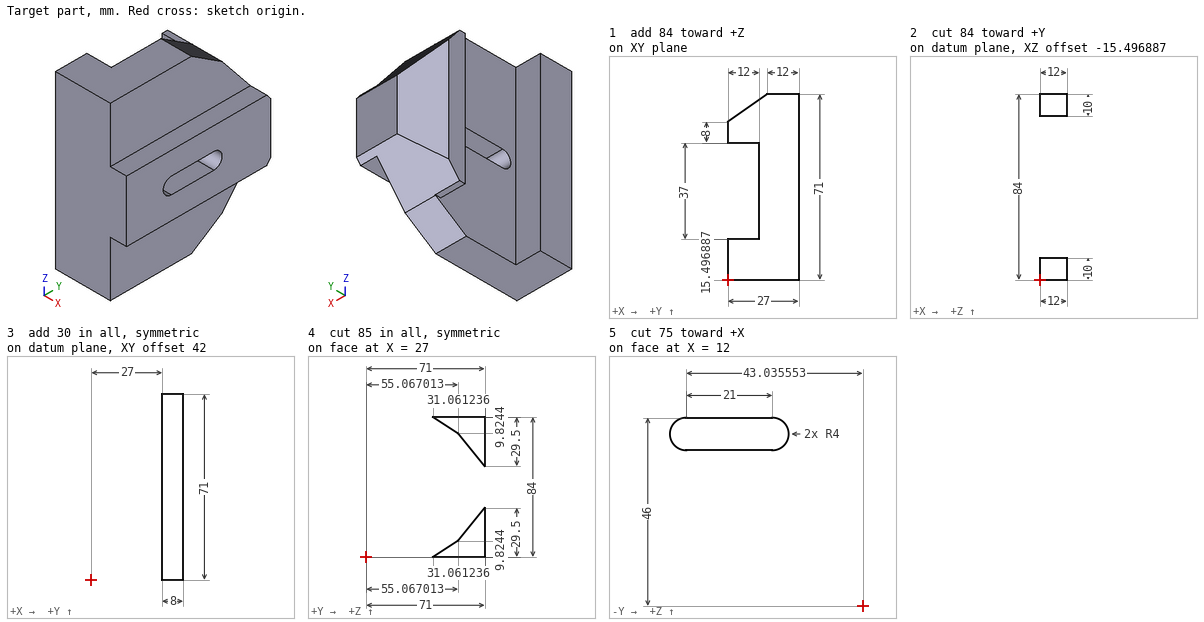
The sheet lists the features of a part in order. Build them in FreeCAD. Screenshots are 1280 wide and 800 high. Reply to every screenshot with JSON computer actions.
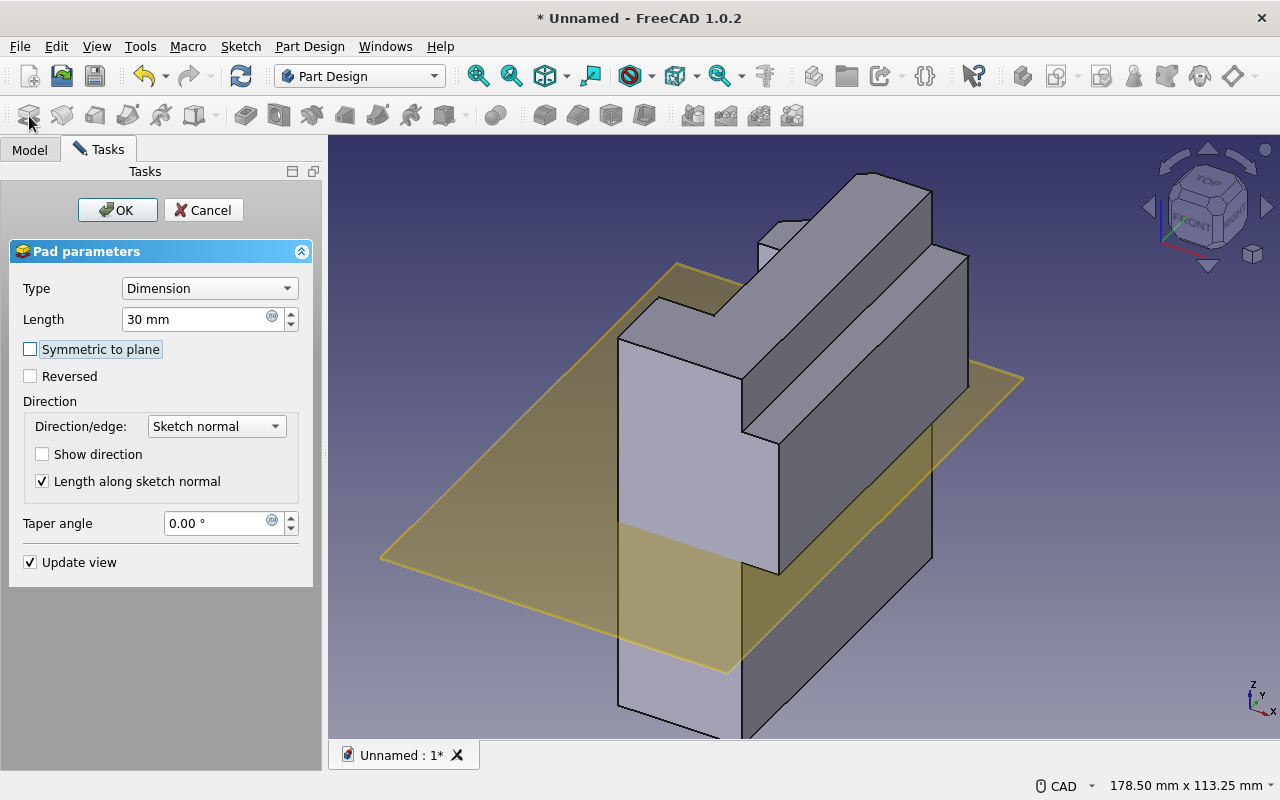
{"action": "left_click", "coordinate": [31, 349]}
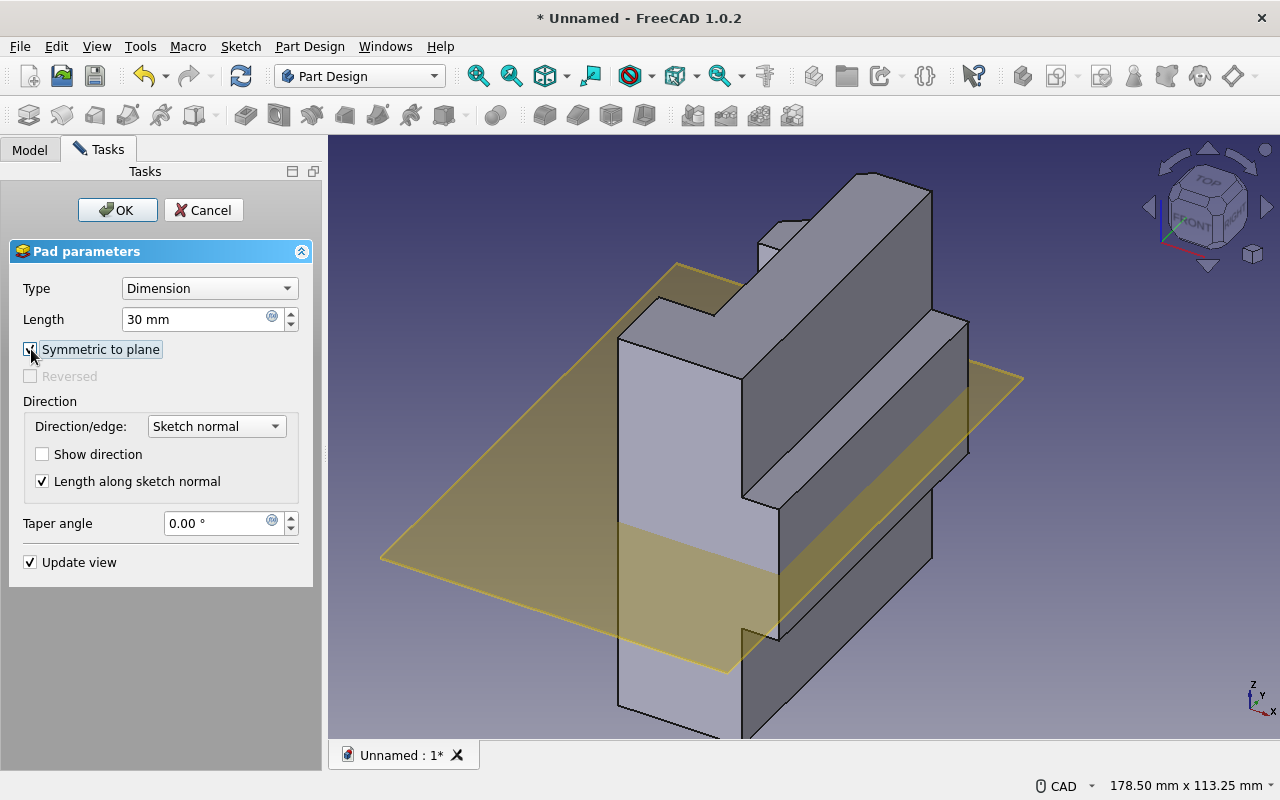
{"action": "left_click", "coordinate": [118, 210]}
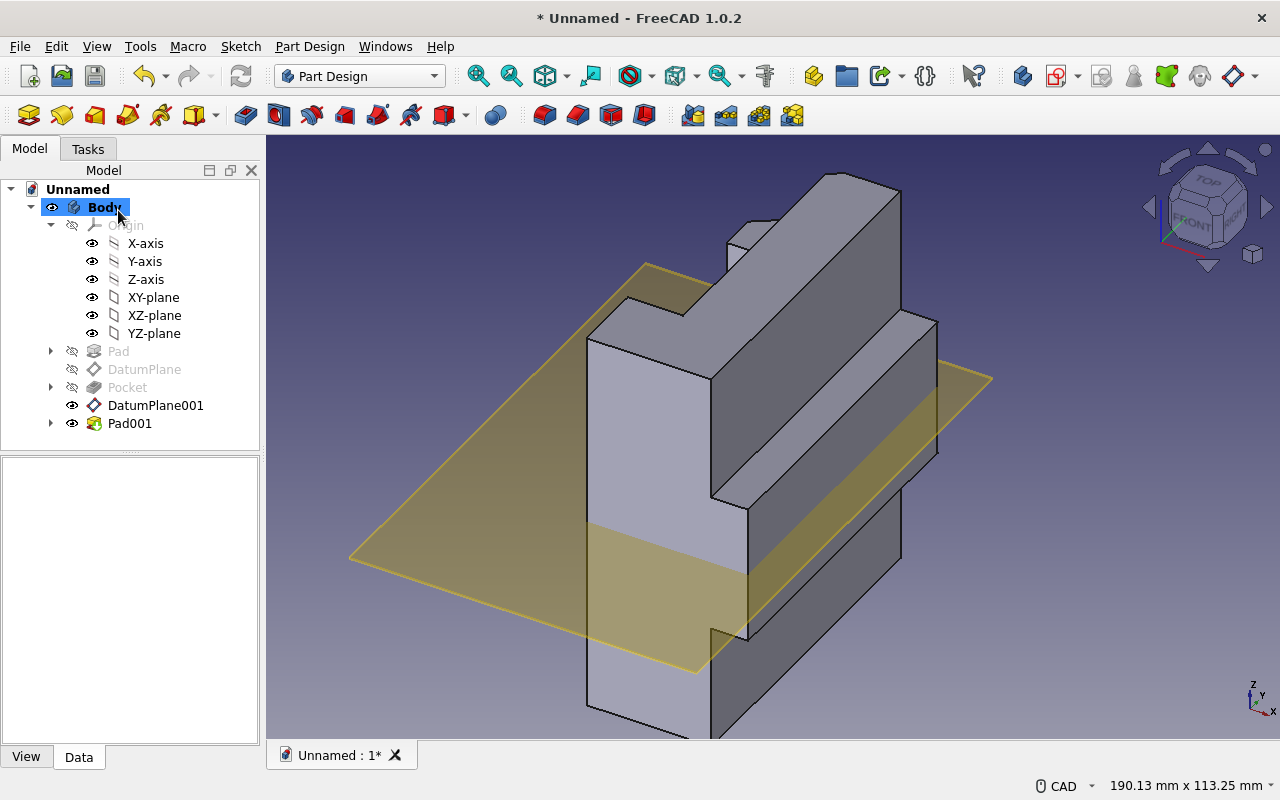
{"action": "left_click", "coordinate": [117, 405]}
{"action": "key", "text": "space"}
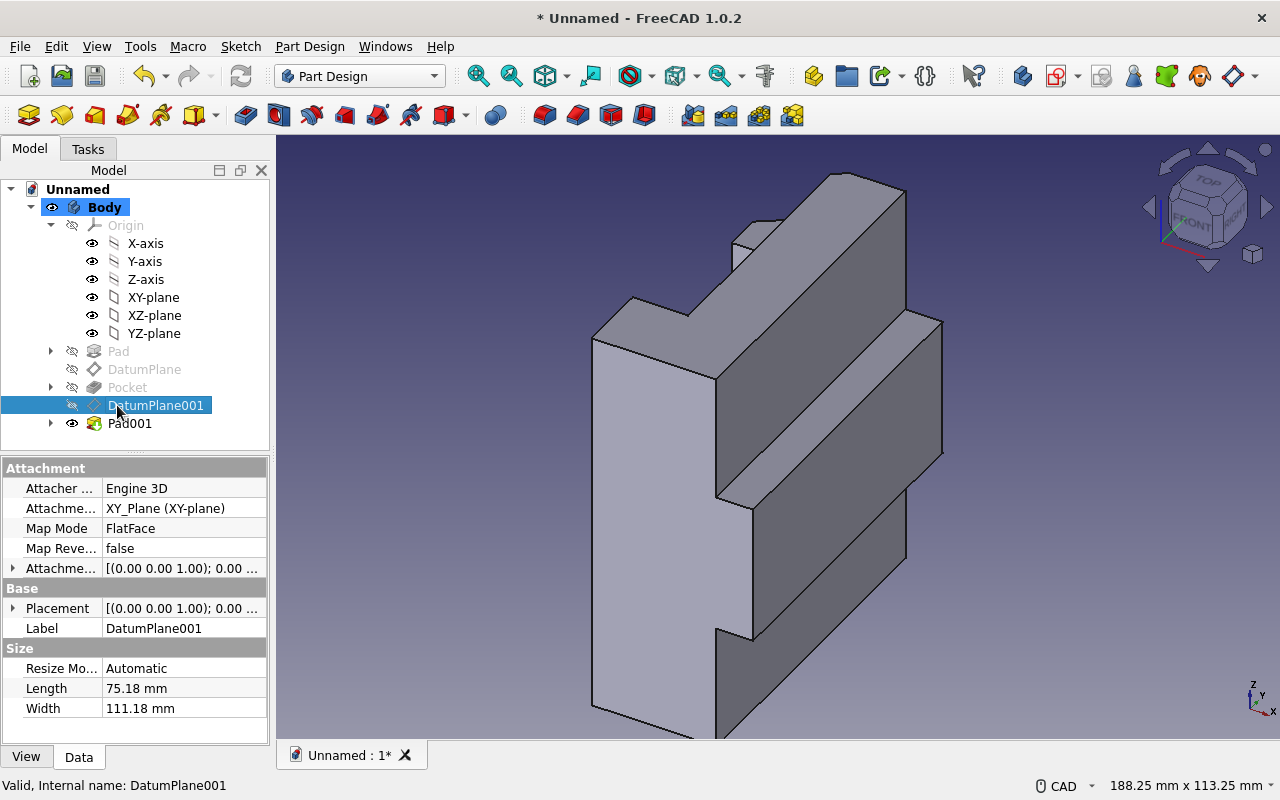
{"action": "left_click", "coordinate": [479, 76]}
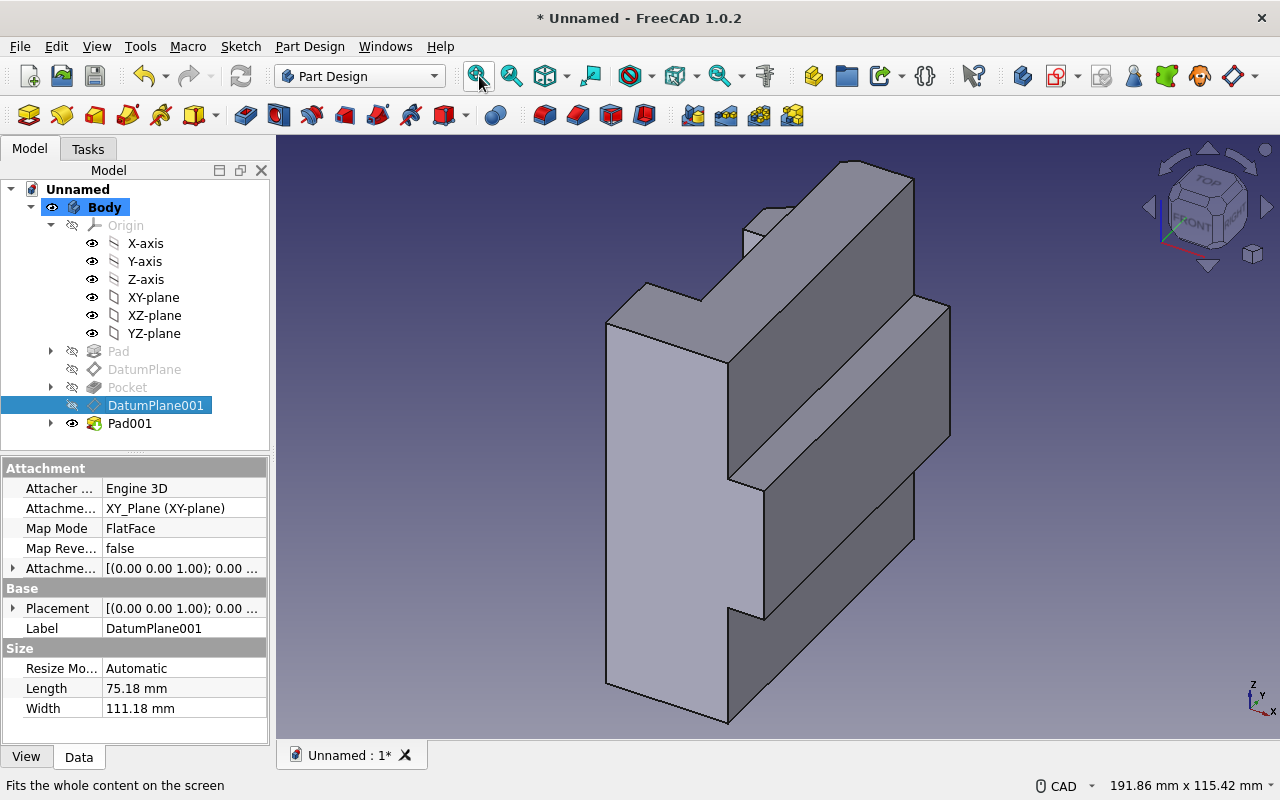
{"action": "left_click", "coordinate": [874, 275]}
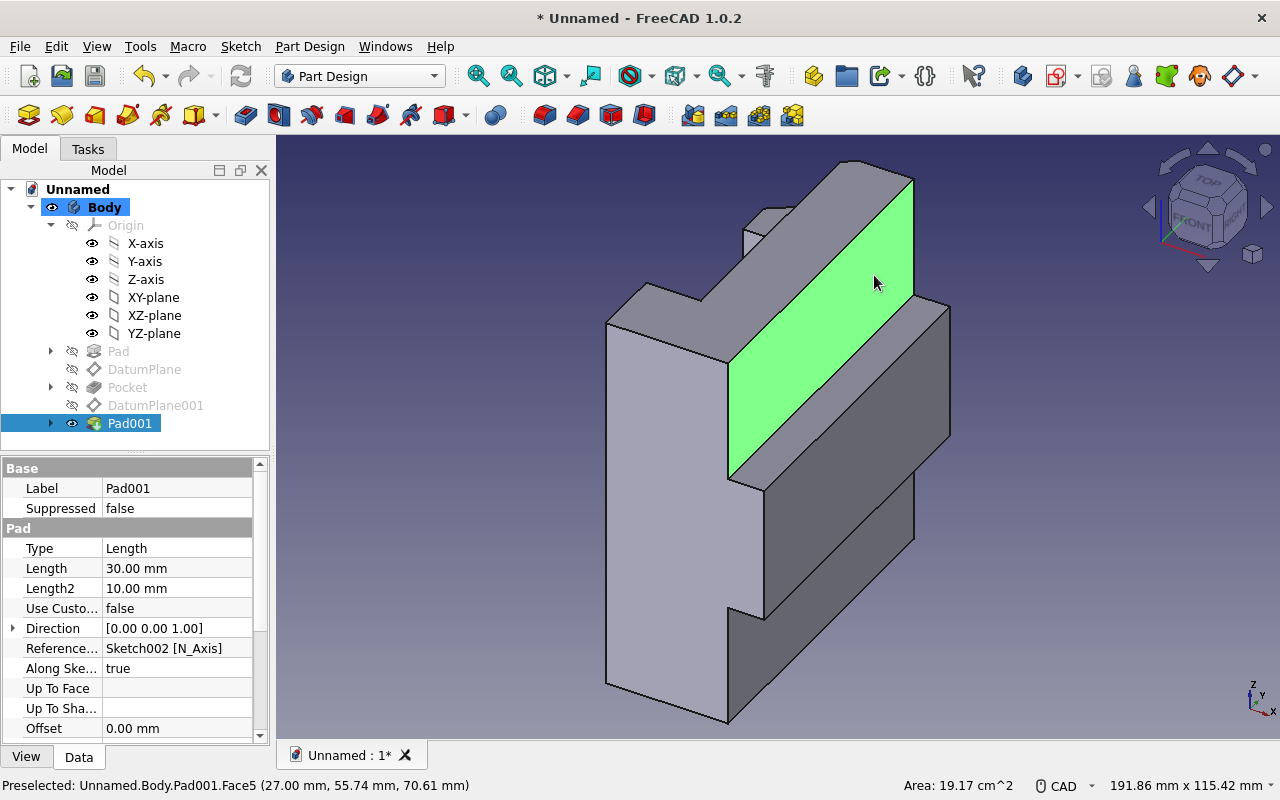
{"action": "left_click", "coordinate": [1056, 76]}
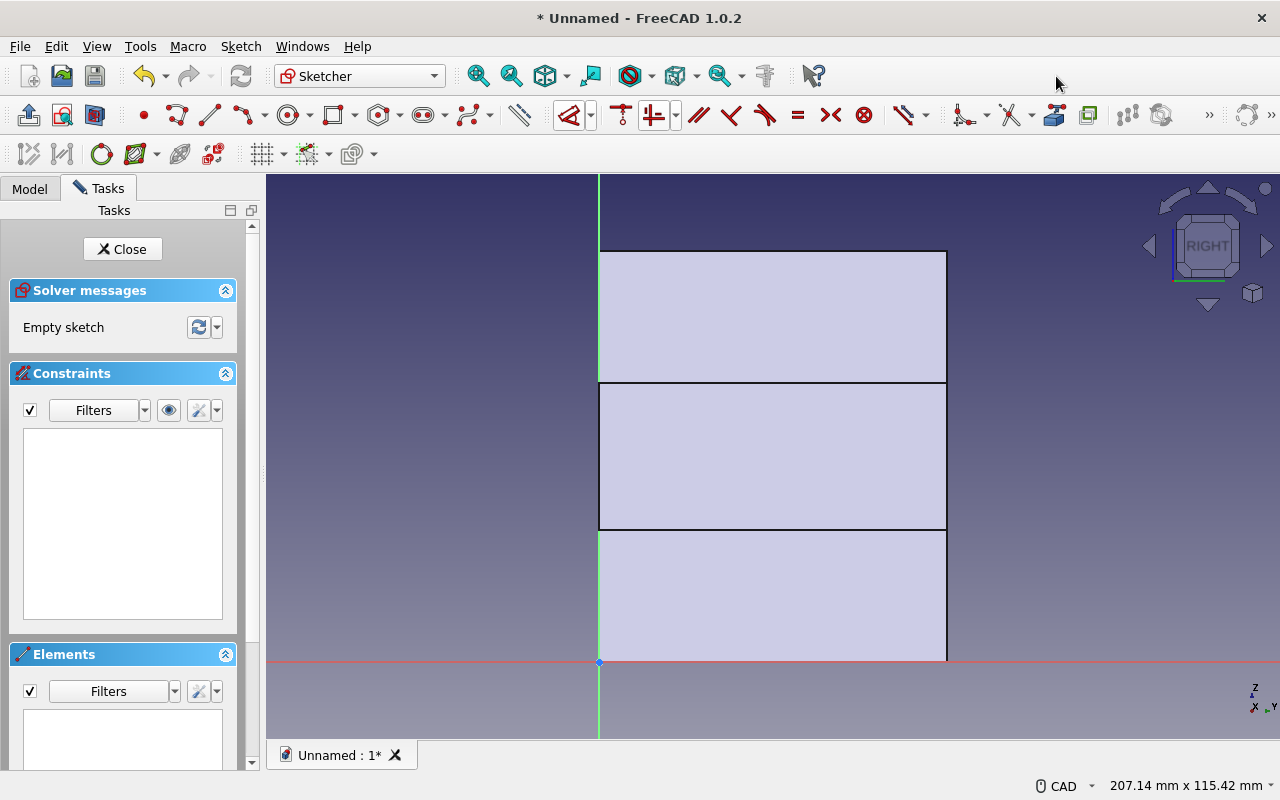
{"action": "key", "text": "q s"}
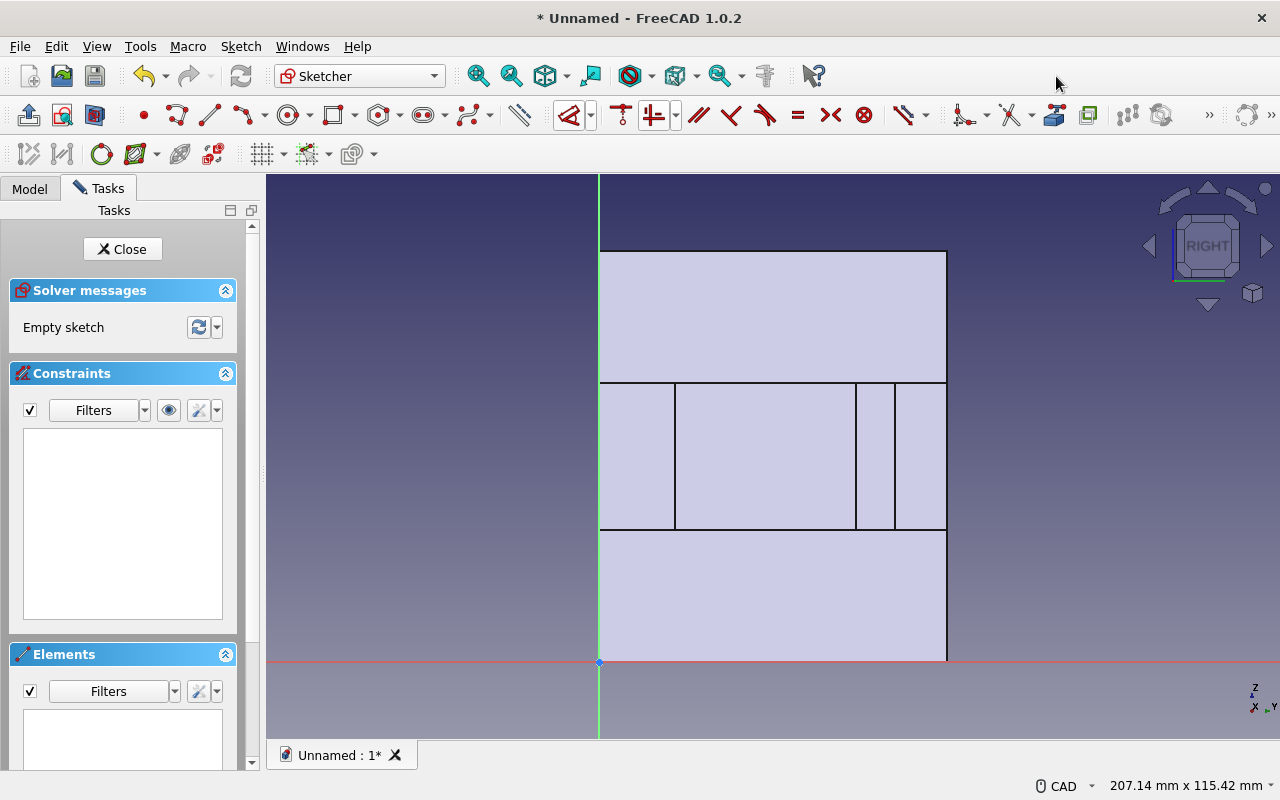
{"action": "key", "text": "g m"}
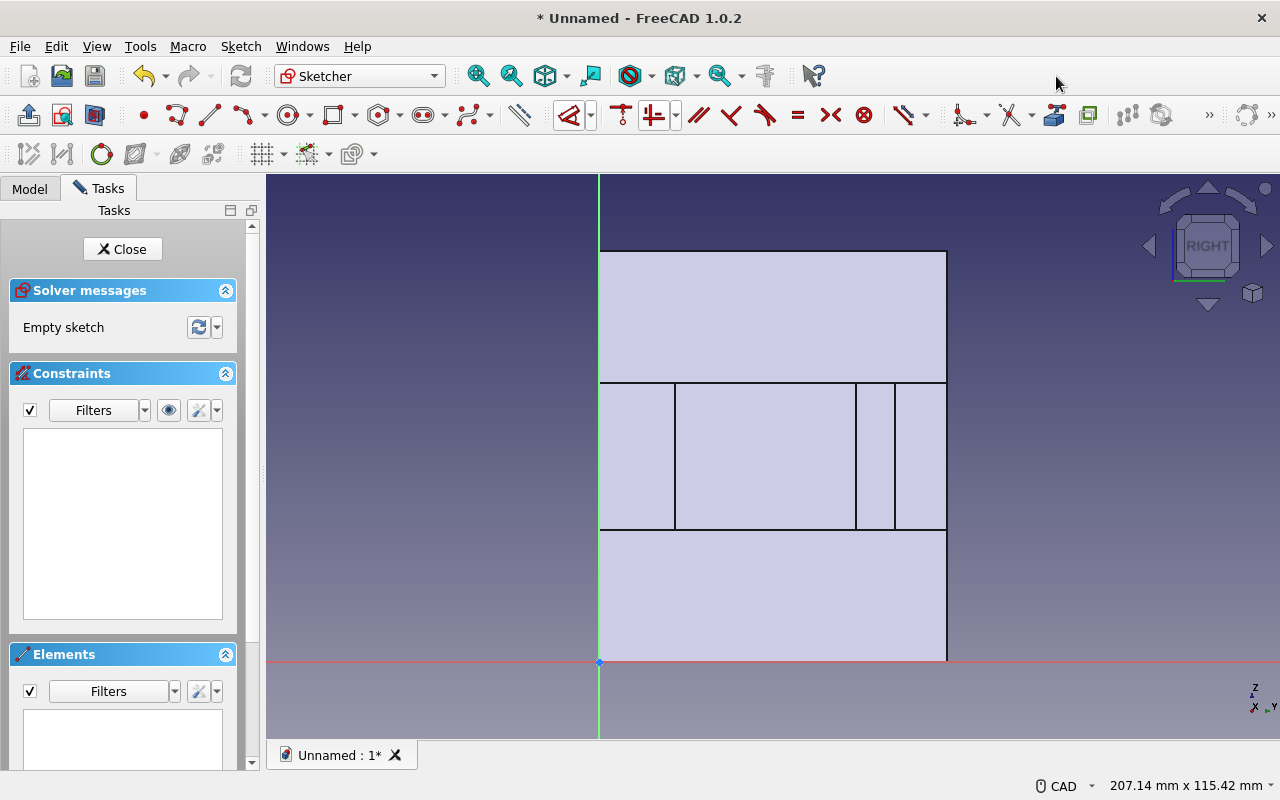
{"action": "left_click", "coordinate": [947, 395]}
{"action": "left_click", "coordinate": [947, 251]}
{"action": "left_click", "coordinate": [795, 251]}
{"action": "left_click", "coordinate": [869, 299]}
{"action": "left_click", "coordinate": [947, 396]}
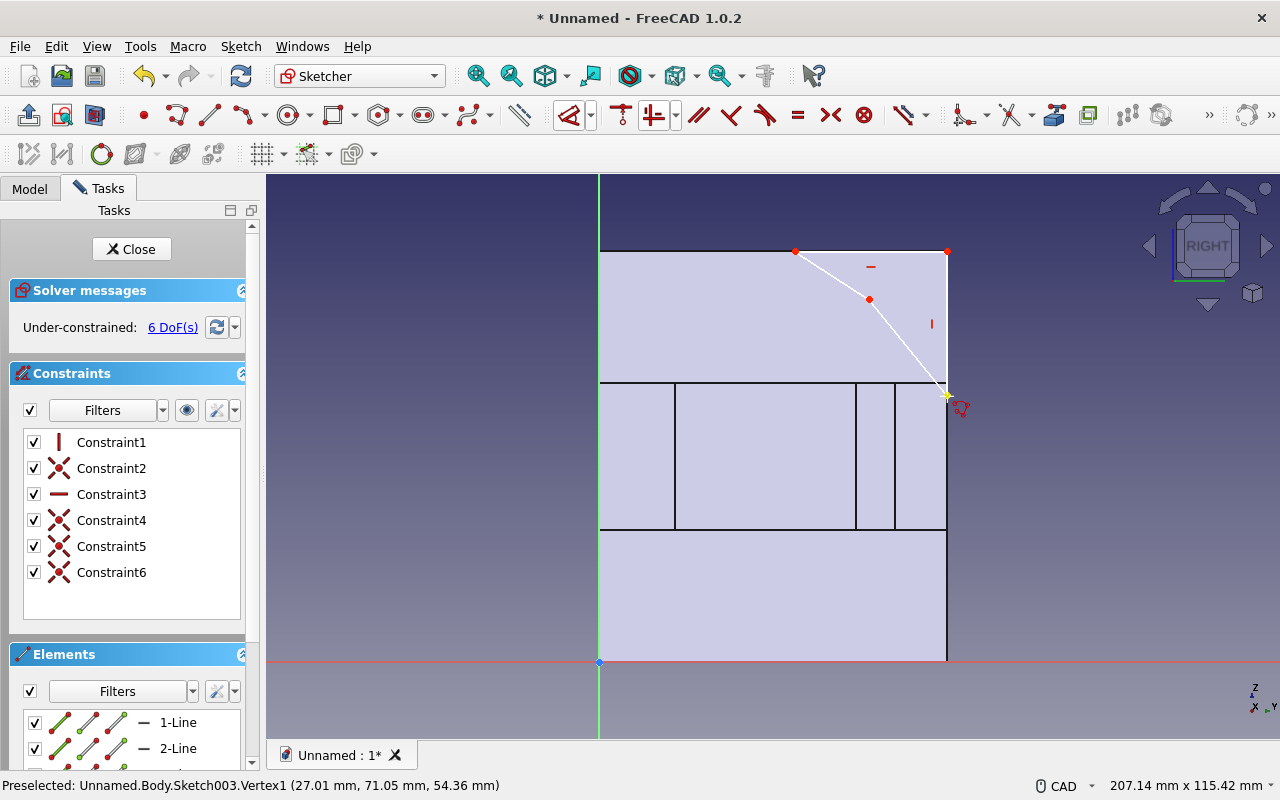
{"action": "left_click", "coordinate": [795, 662]}
{"action": "left_click", "coordinate": [947, 653]}
{"action": "left_click", "coordinate": [947, 518]}
{"action": "left_click", "coordinate": [869, 614]}
{"action": "left_click", "coordinate": [795, 662]}
{"action": "key", "text": "Escape"}
{"action": "key", "text": "Escape"}